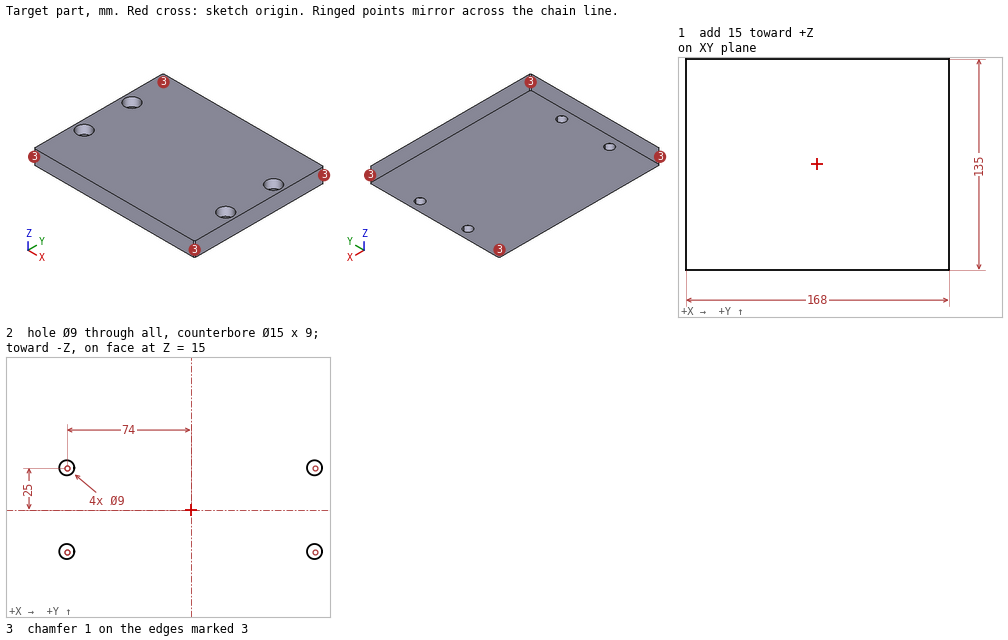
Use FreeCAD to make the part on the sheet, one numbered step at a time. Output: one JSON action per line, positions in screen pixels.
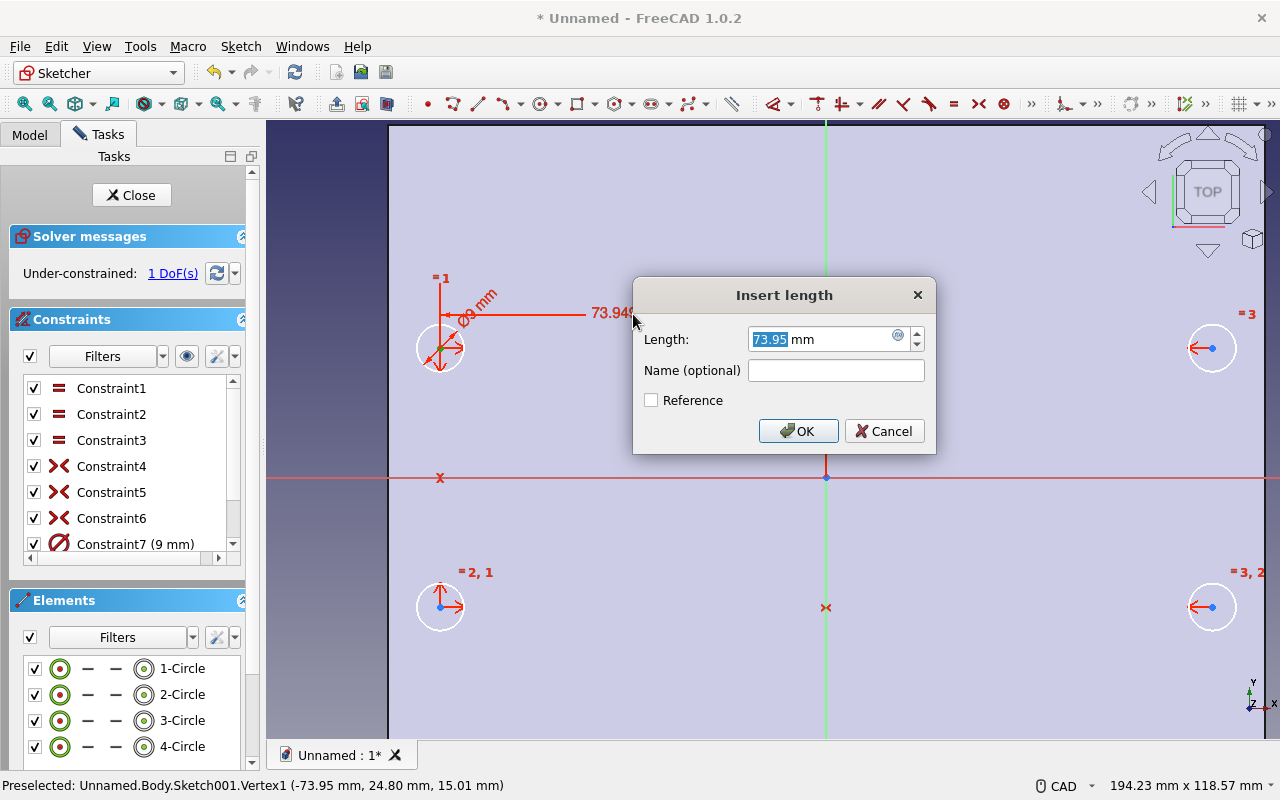
{"action": "type", "text": "74"}
{"action": "key", "text": "Return"}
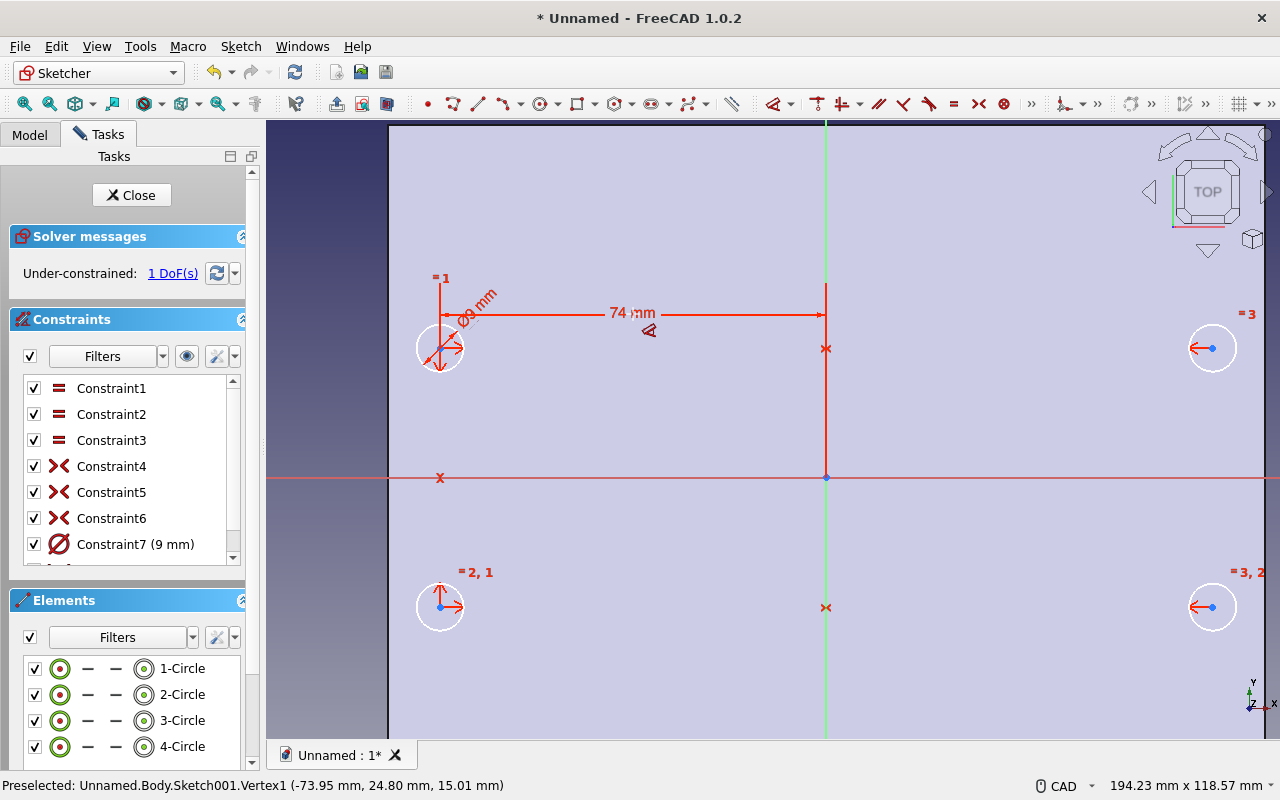
{"action": "left_click", "coordinate": [440, 348]}
{"action": "left_click", "coordinate": [406, 413]}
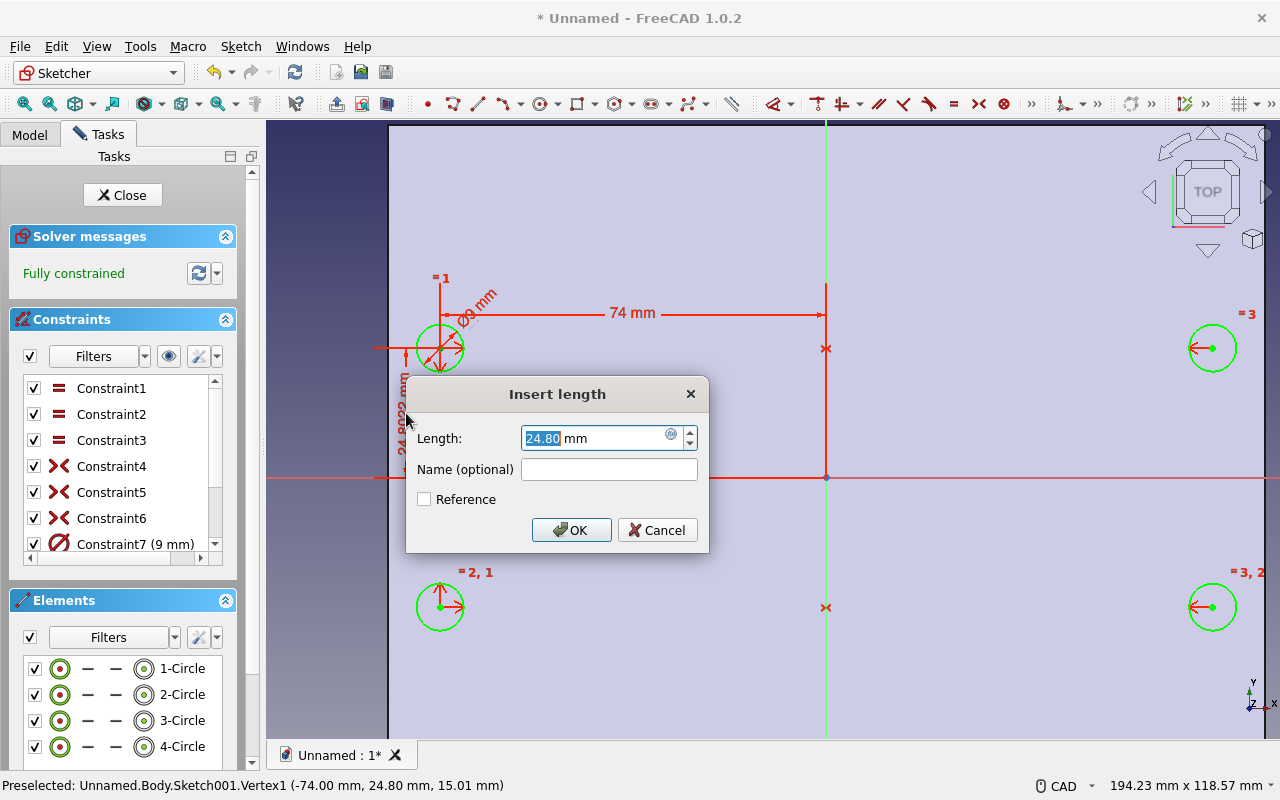
{"action": "type", "text": "25"}
{"action": "key", "text": "Return"}
{"action": "key", "text": "Escape"}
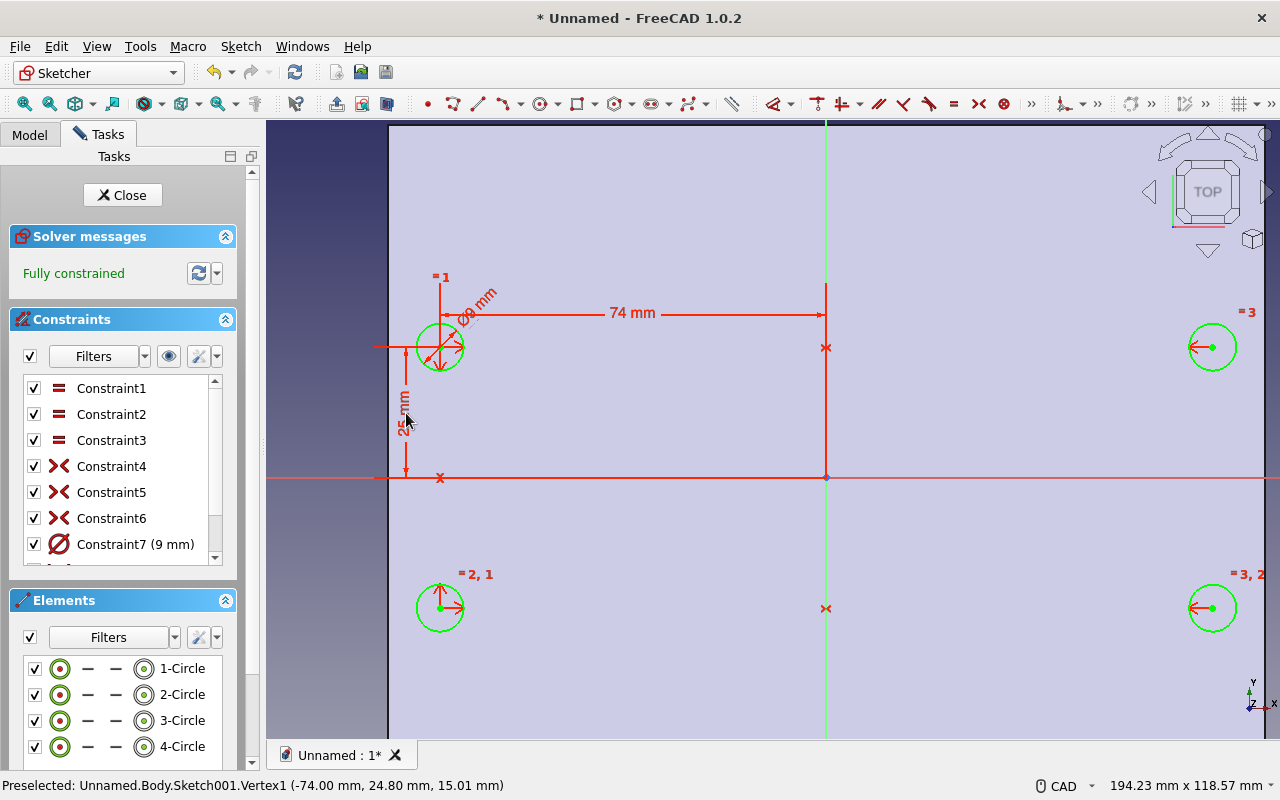
{"action": "left_click", "coordinate": [123, 195]}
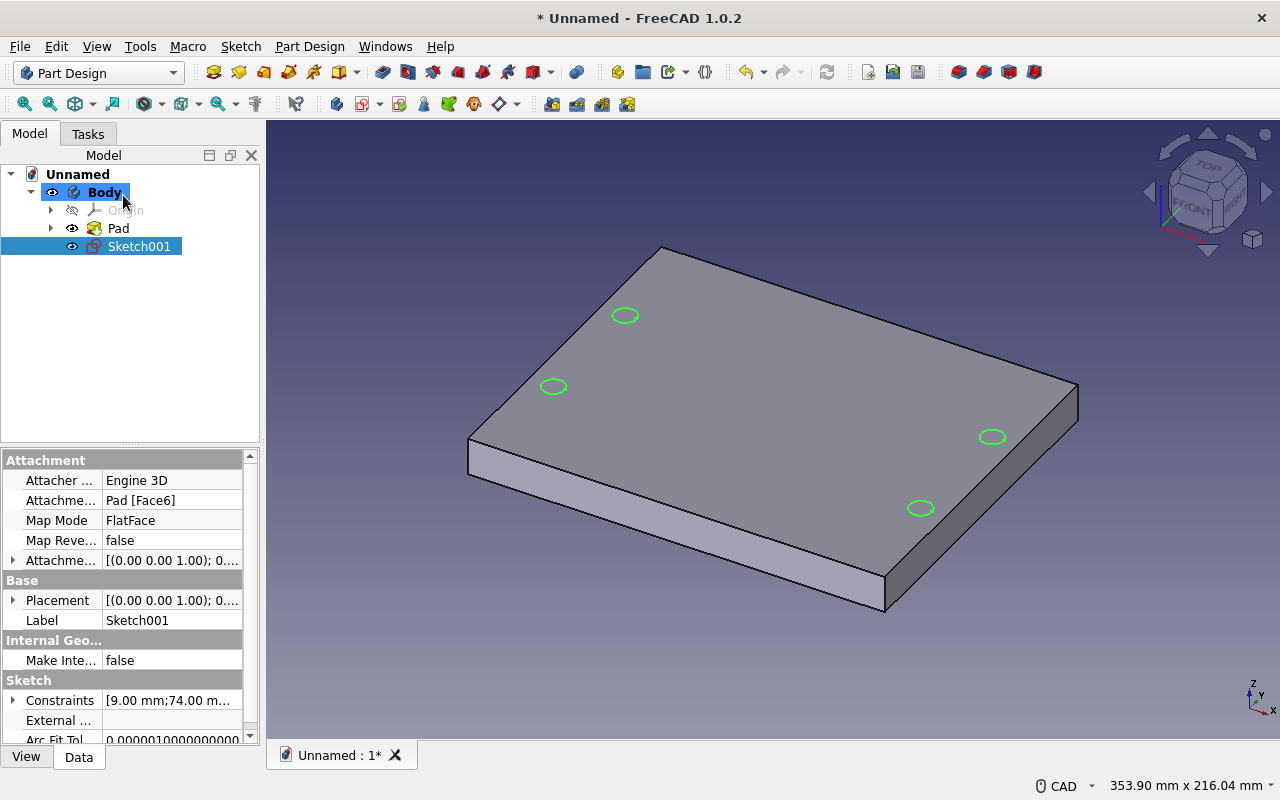
{"action": "left_click", "coordinate": [408, 72]}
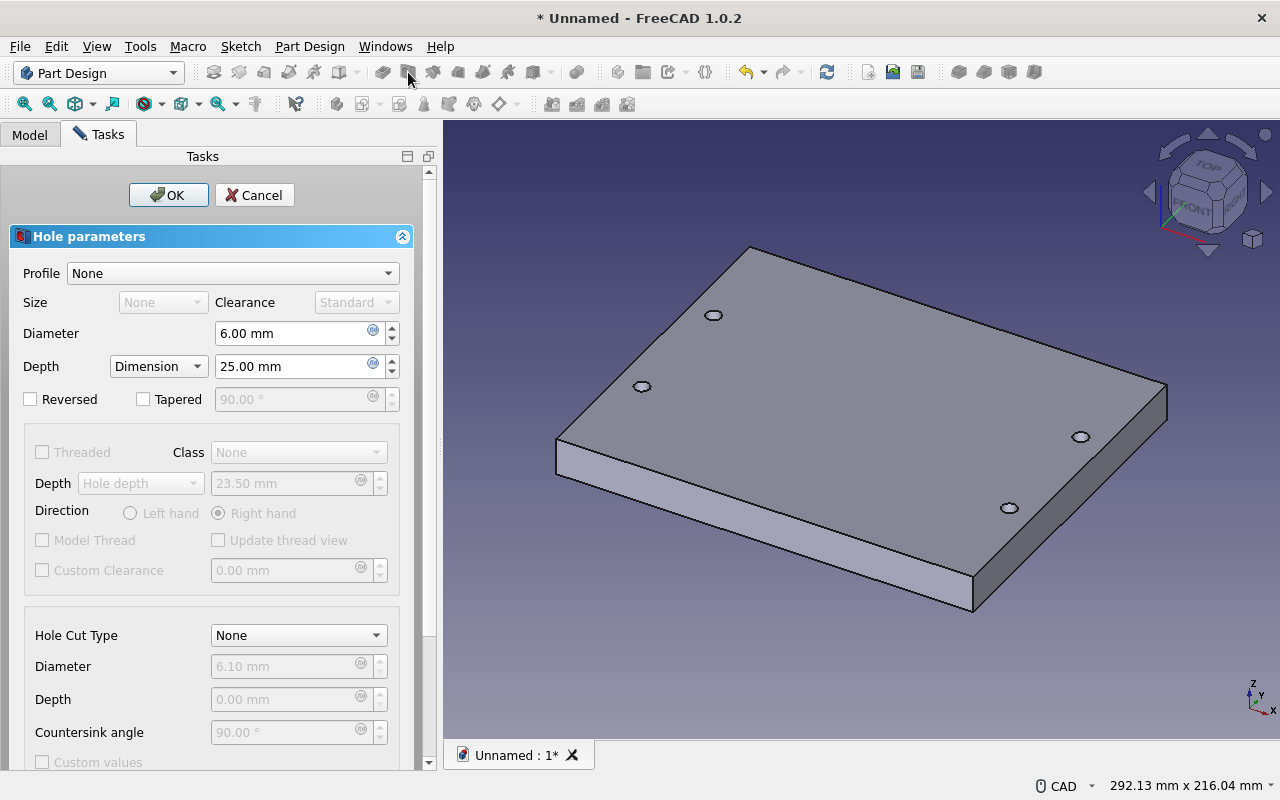
{"action": "triple_click", "coordinate": [300, 334]}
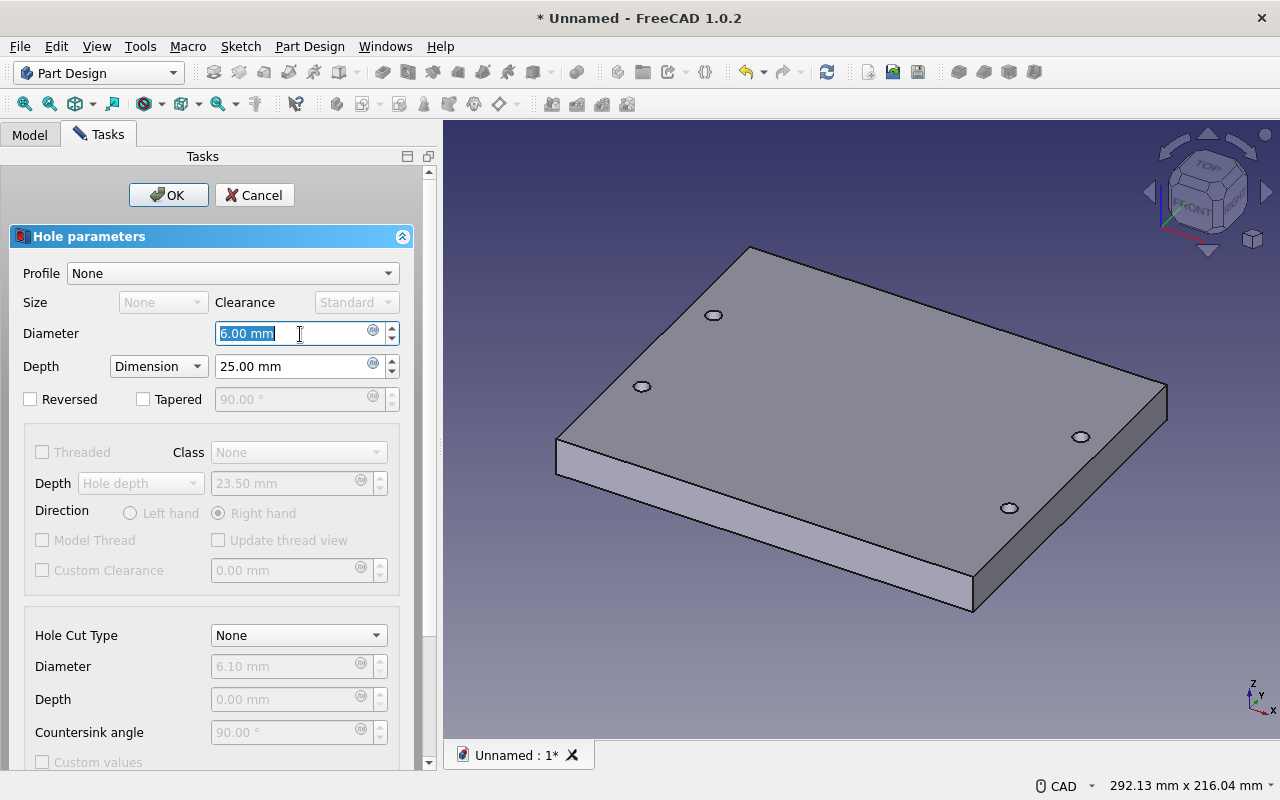
{"action": "type", "text": "9"}
{"action": "key", "text": "Tab"}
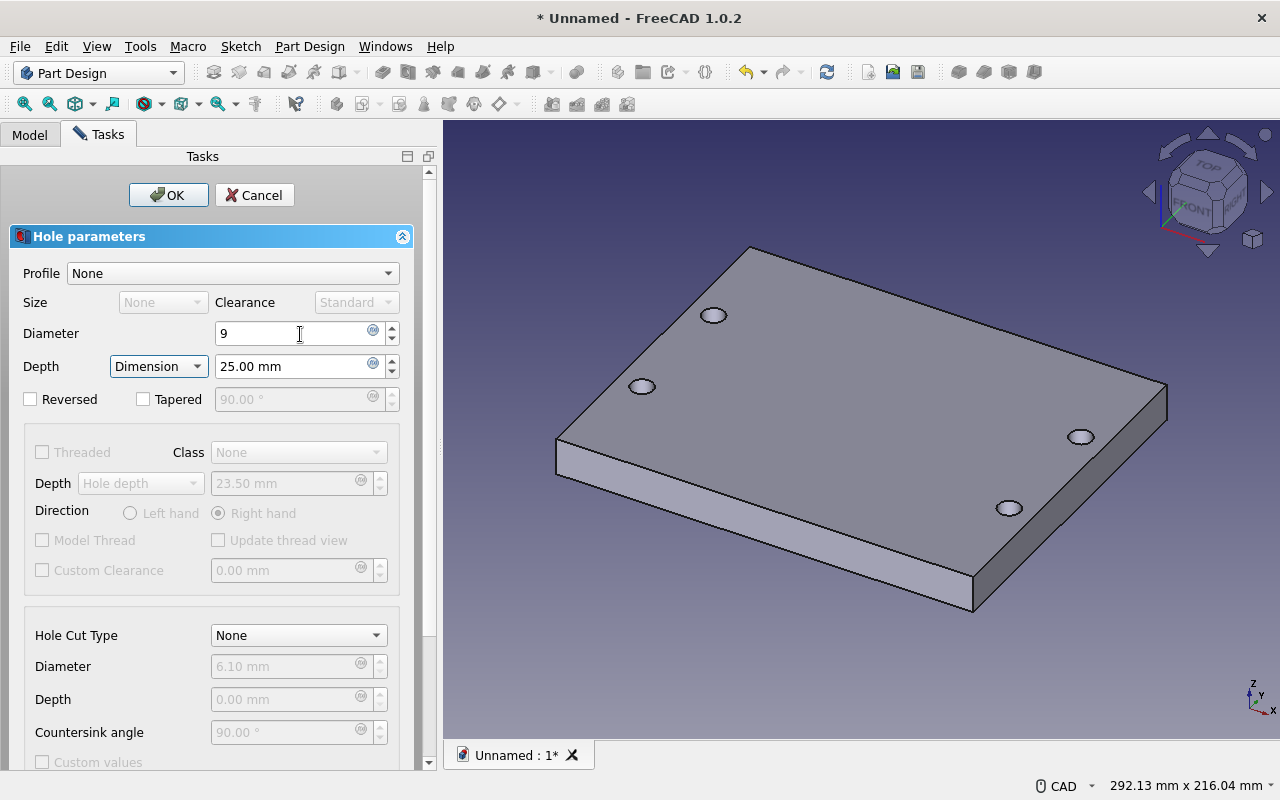
{"action": "left_click", "coordinate": [160, 366]}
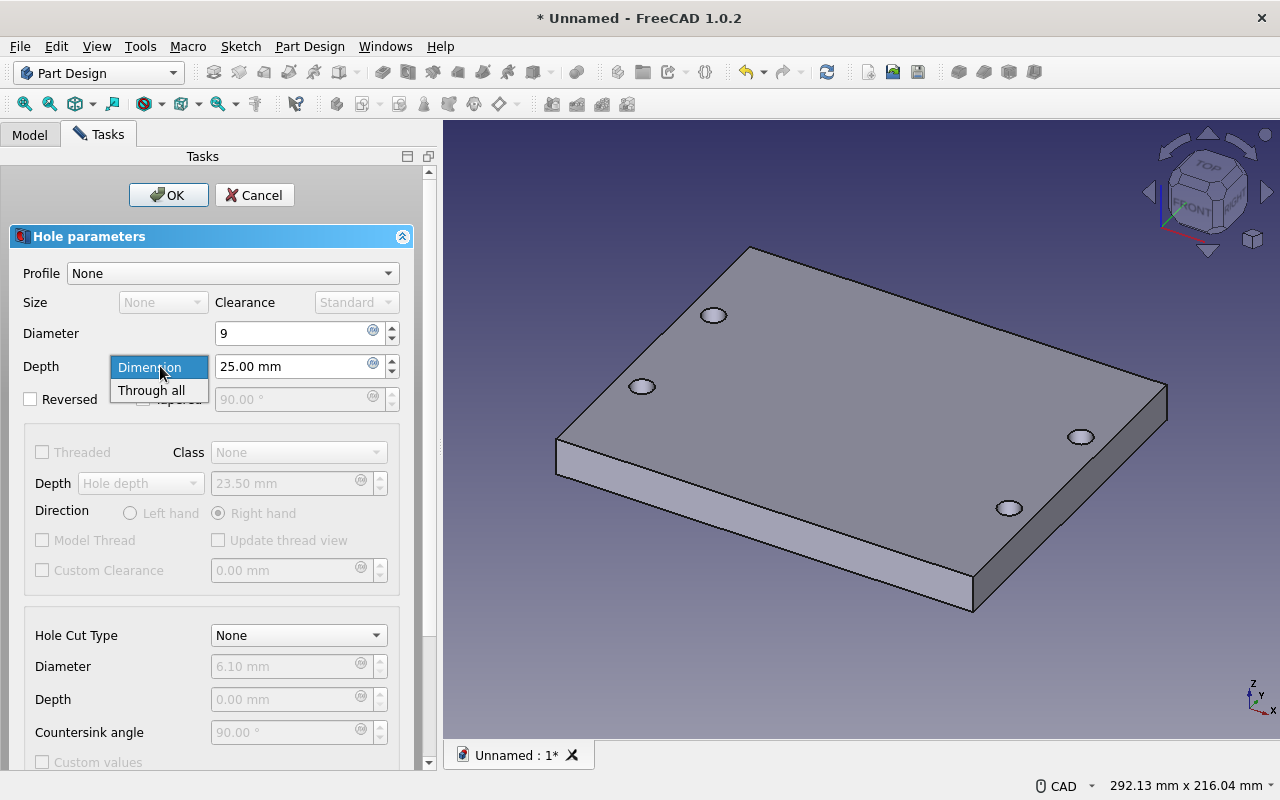
{"action": "left_click", "coordinate": [158, 390]}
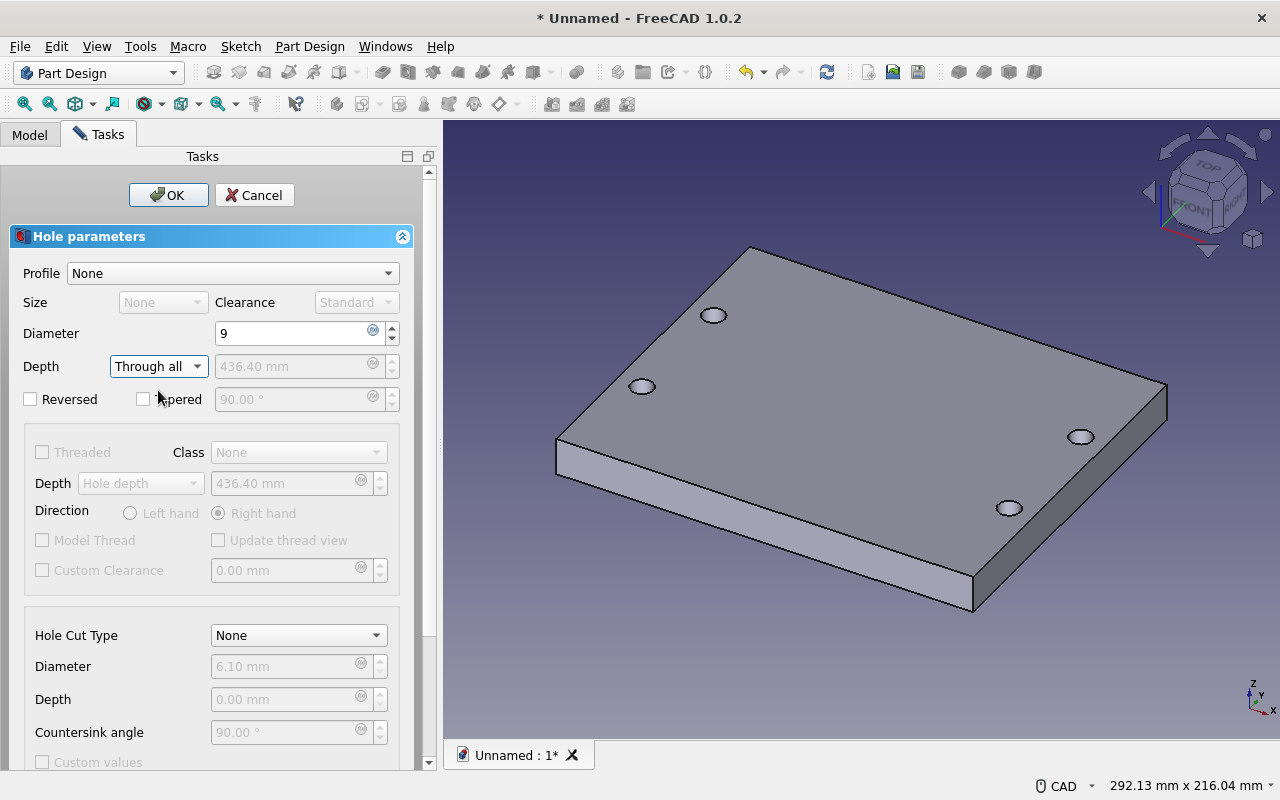
{"action": "left_click", "coordinate": [300, 636]}